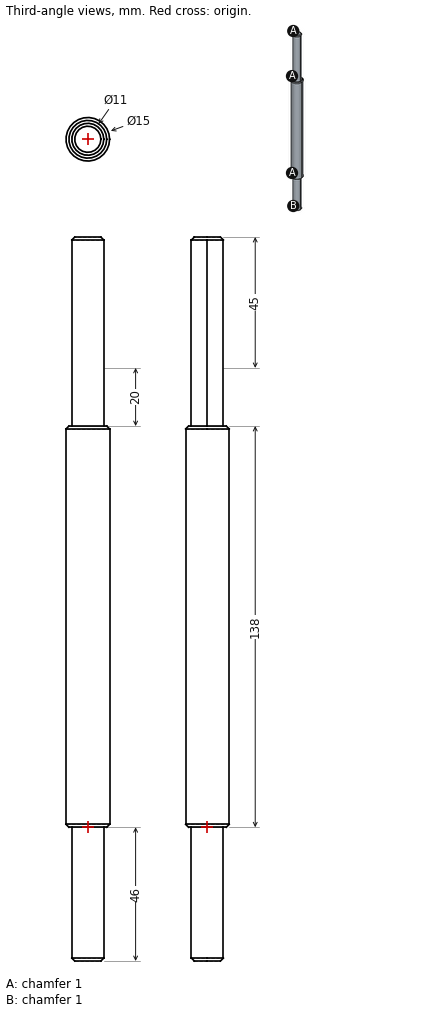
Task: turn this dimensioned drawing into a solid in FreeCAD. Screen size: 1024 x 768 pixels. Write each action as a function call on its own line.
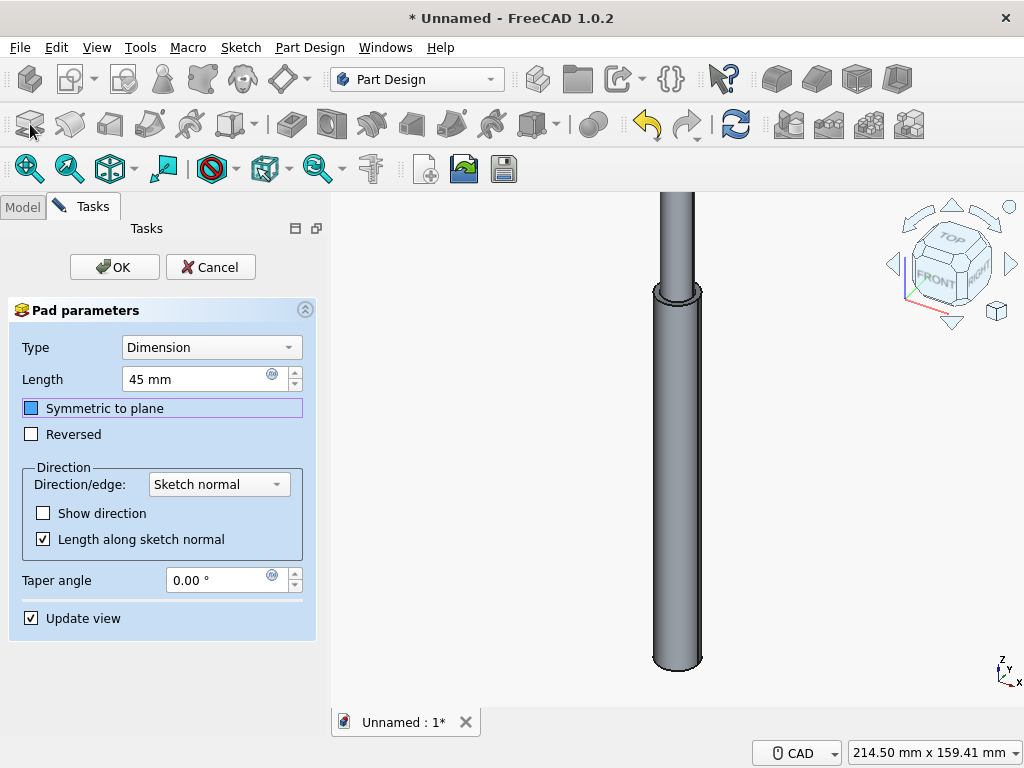
click(115, 267)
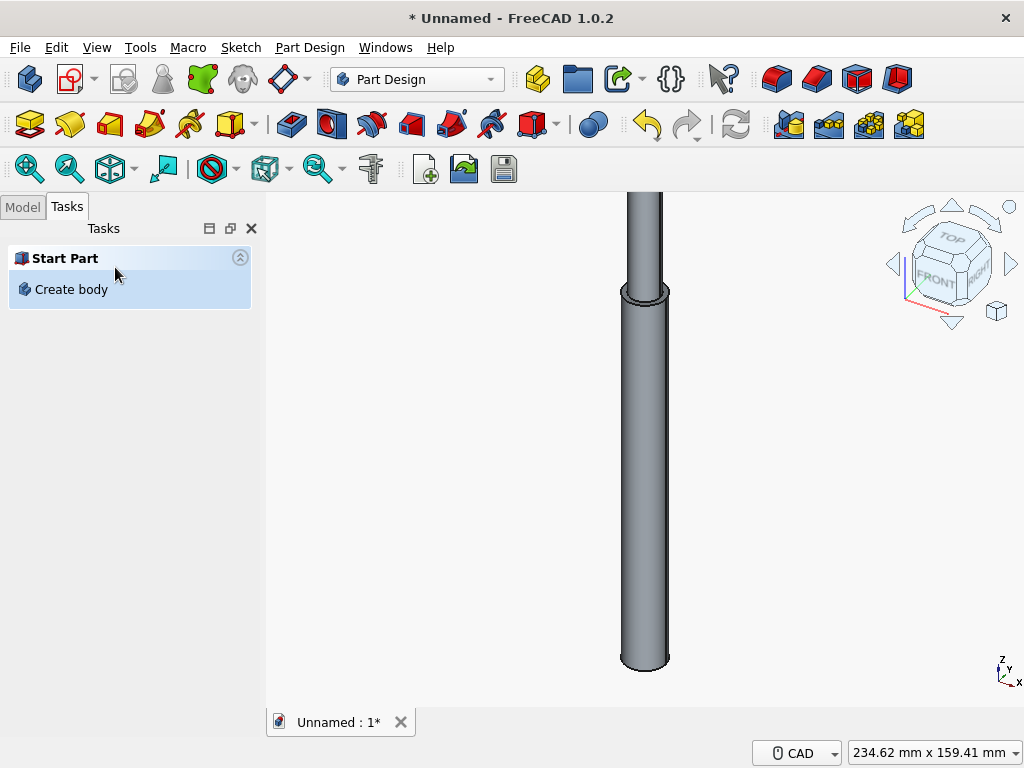
click(30, 170)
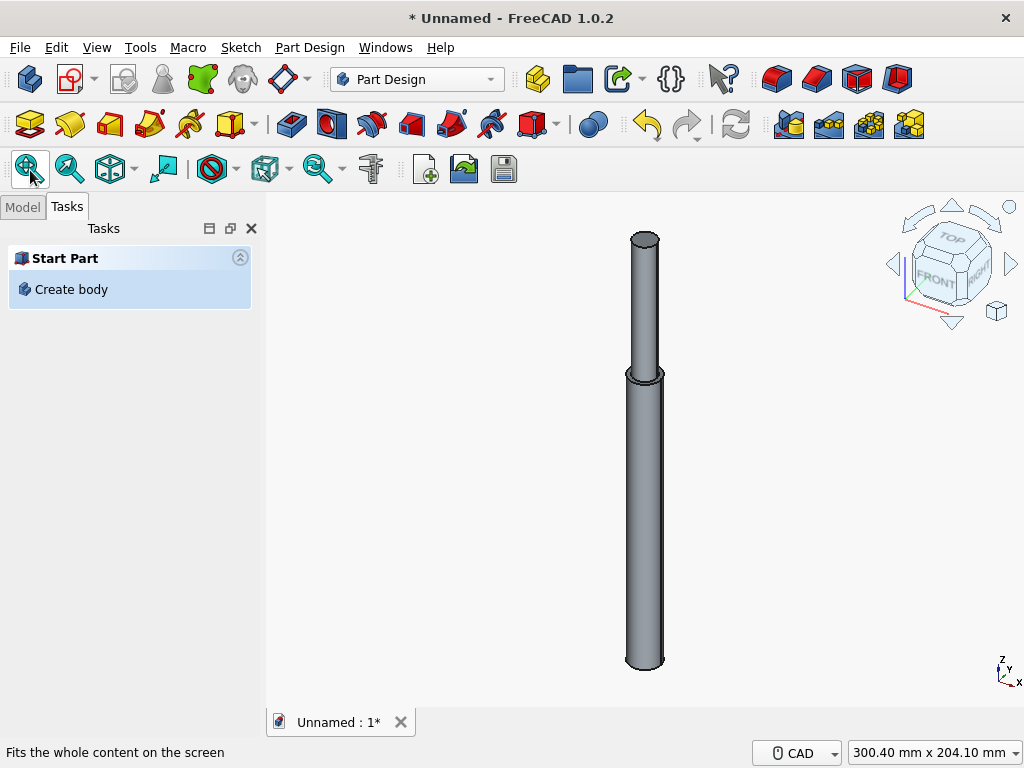
click(631, 666)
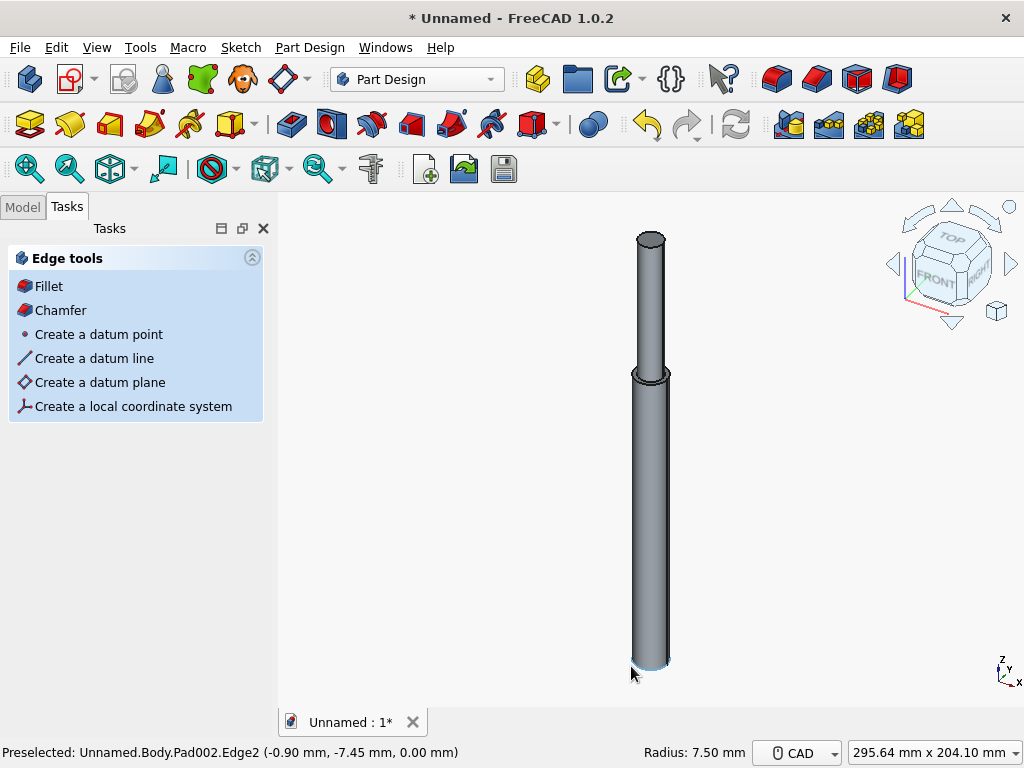
click(632, 374, ctrl)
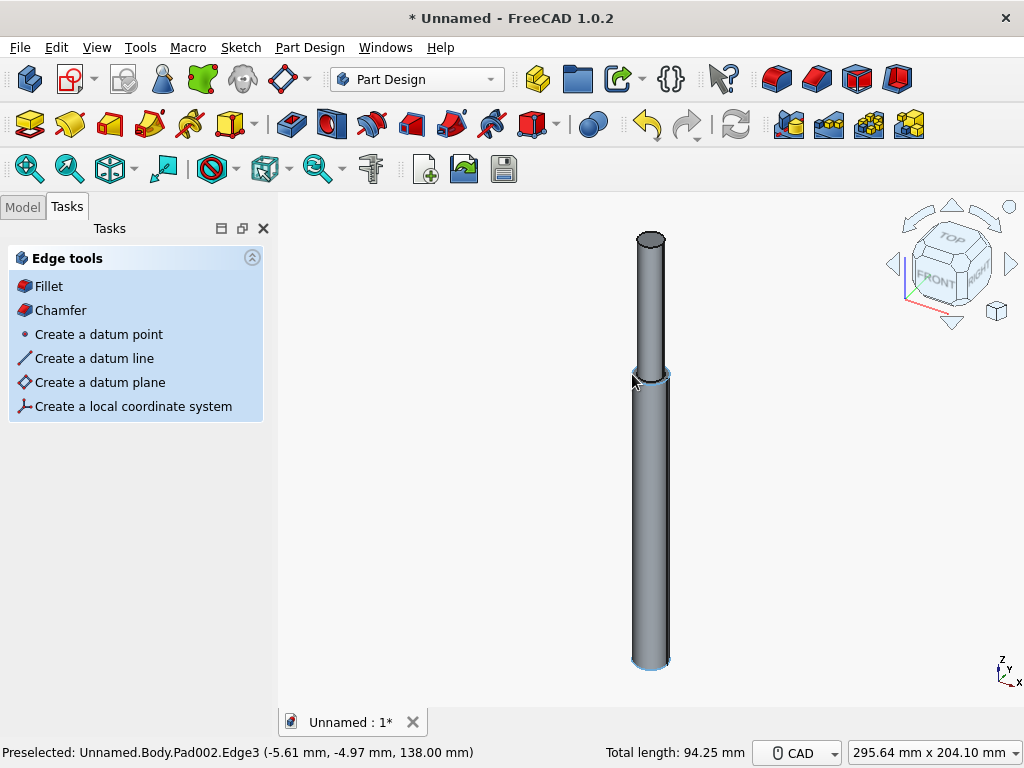
click(639, 235, ctrl)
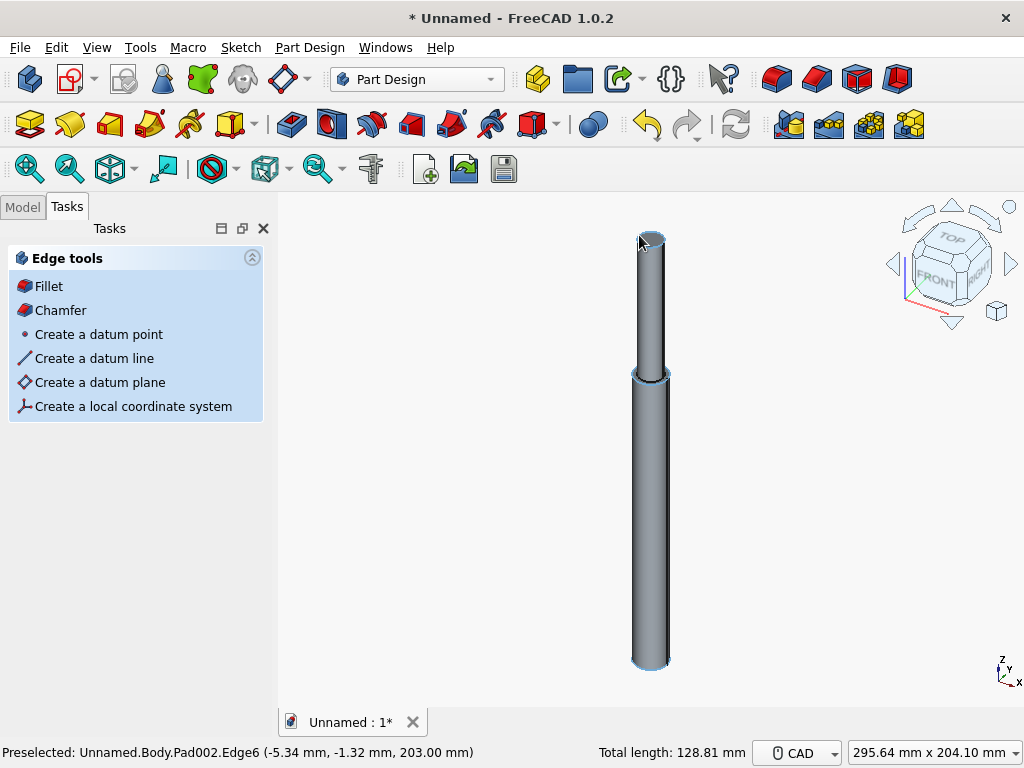
click(818, 80)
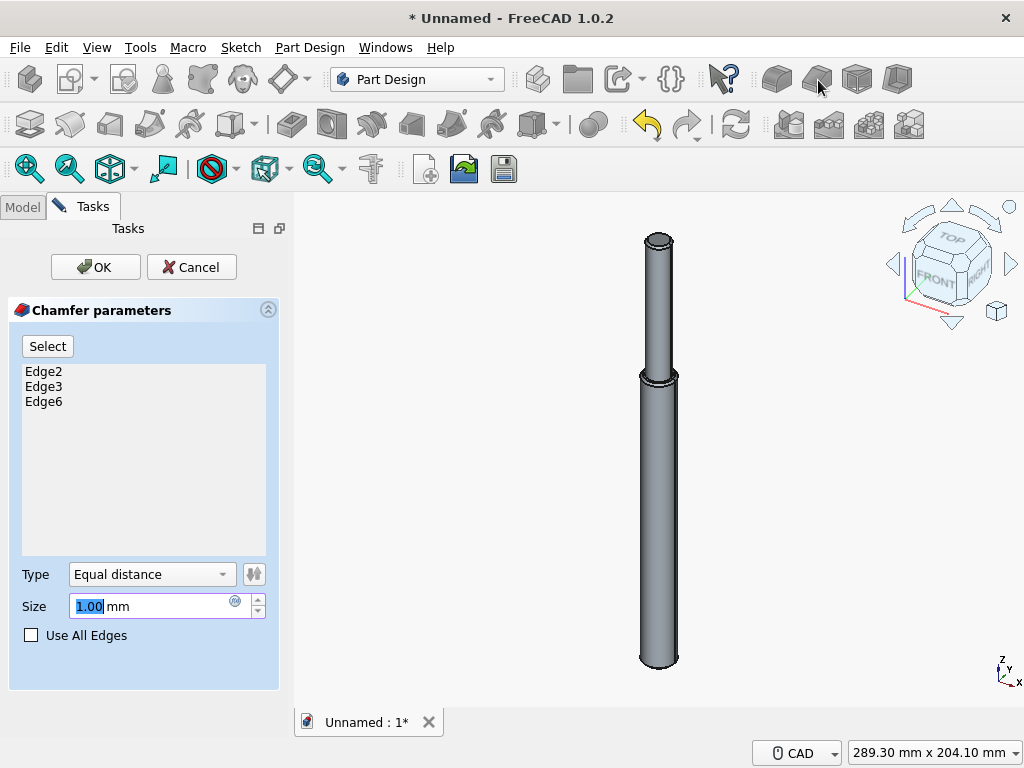
text(1)
key(Tab)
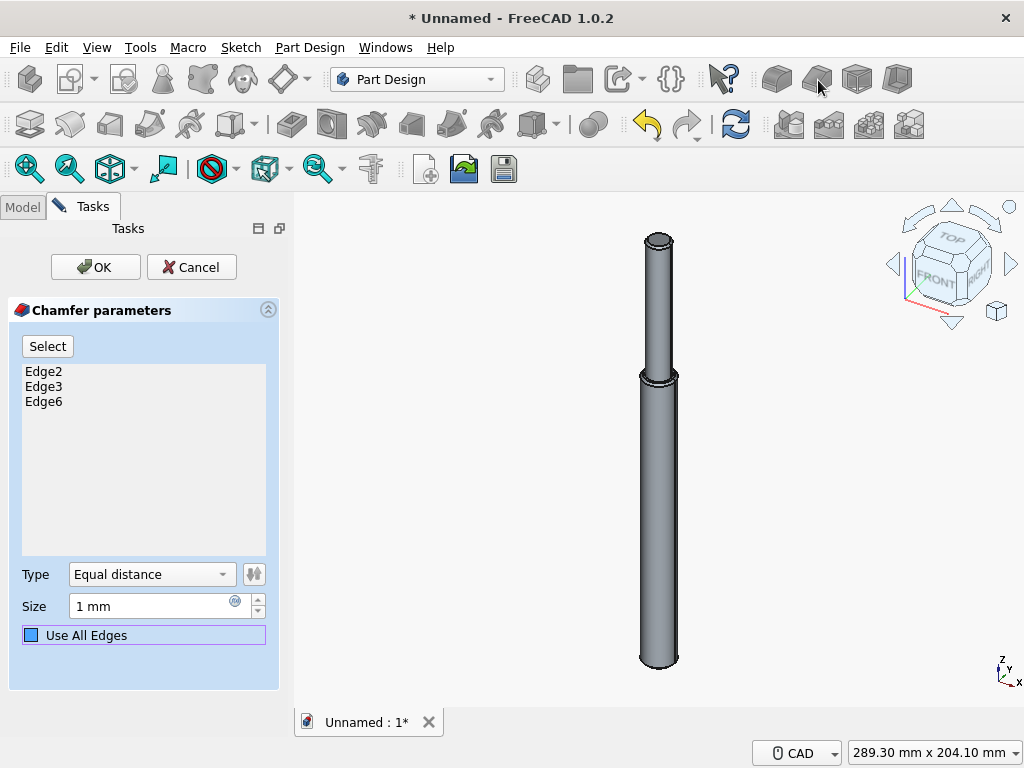
click(96, 267)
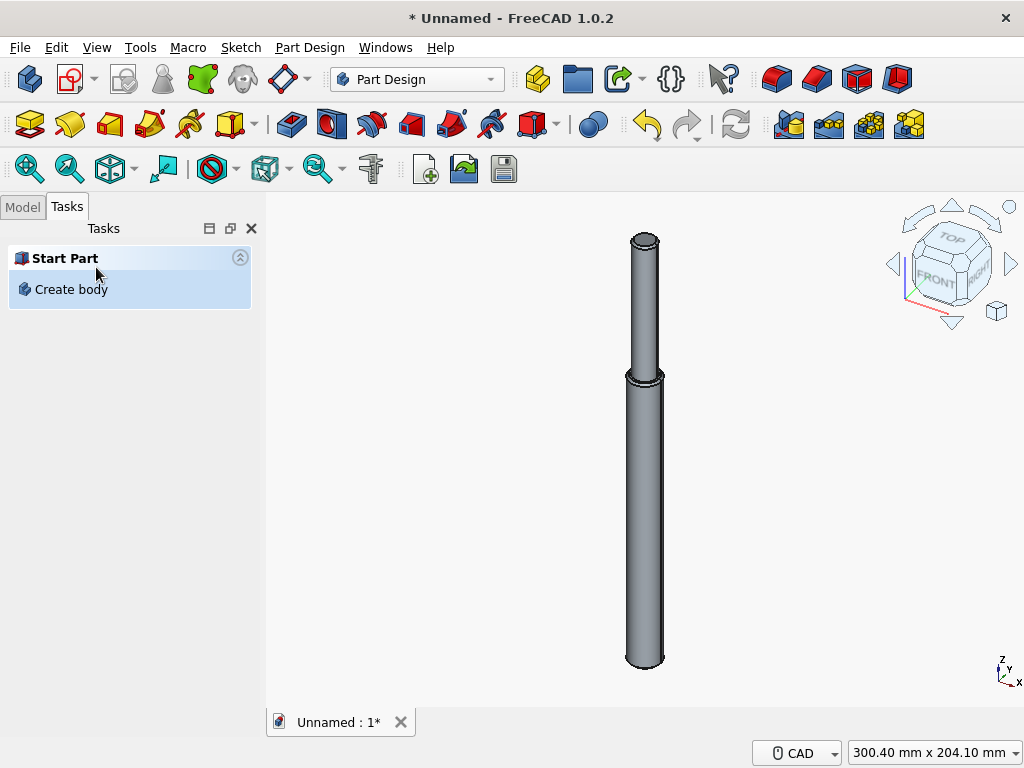
click(23, 206)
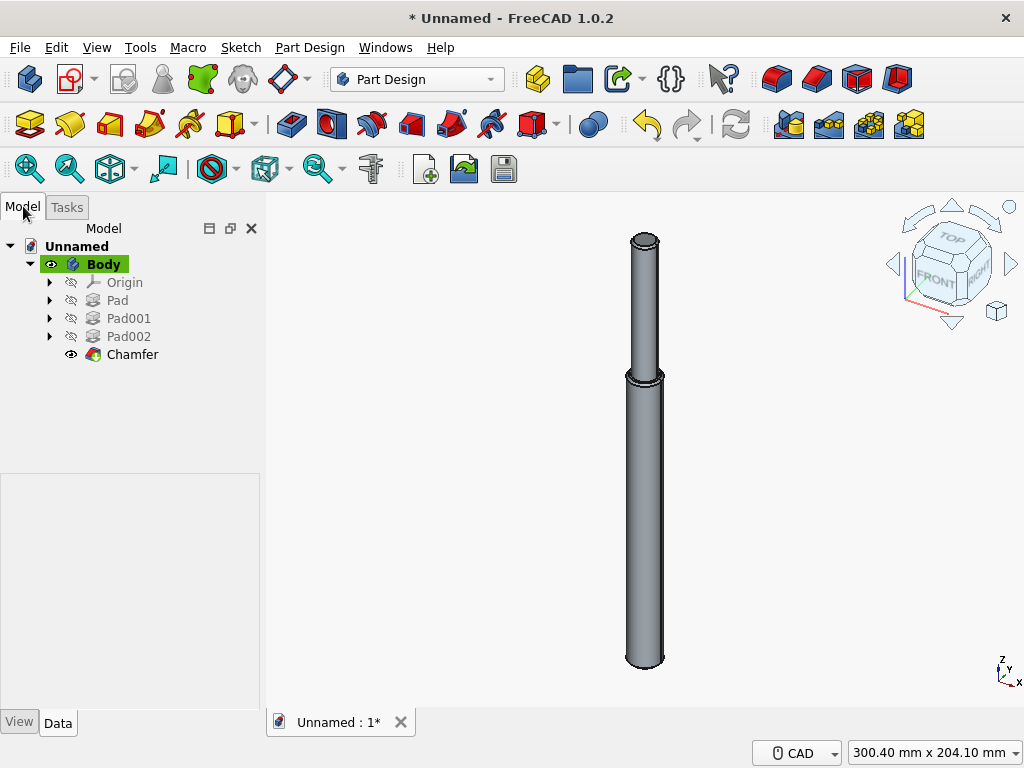
click(50, 282)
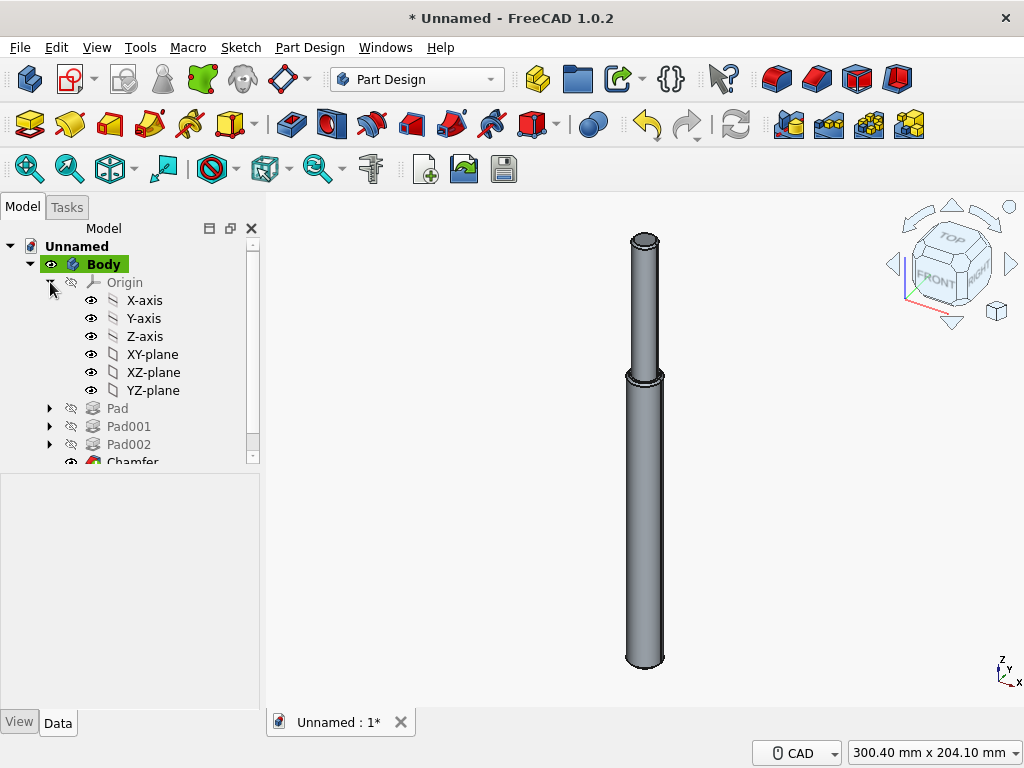
click(136, 354)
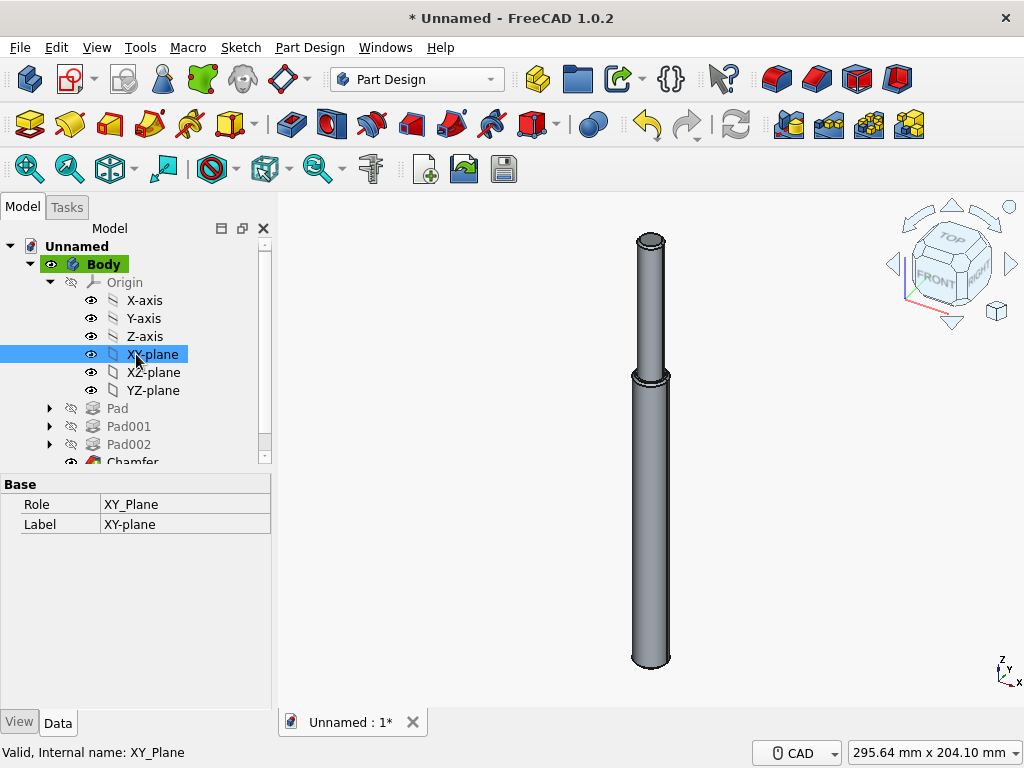
click(284, 80)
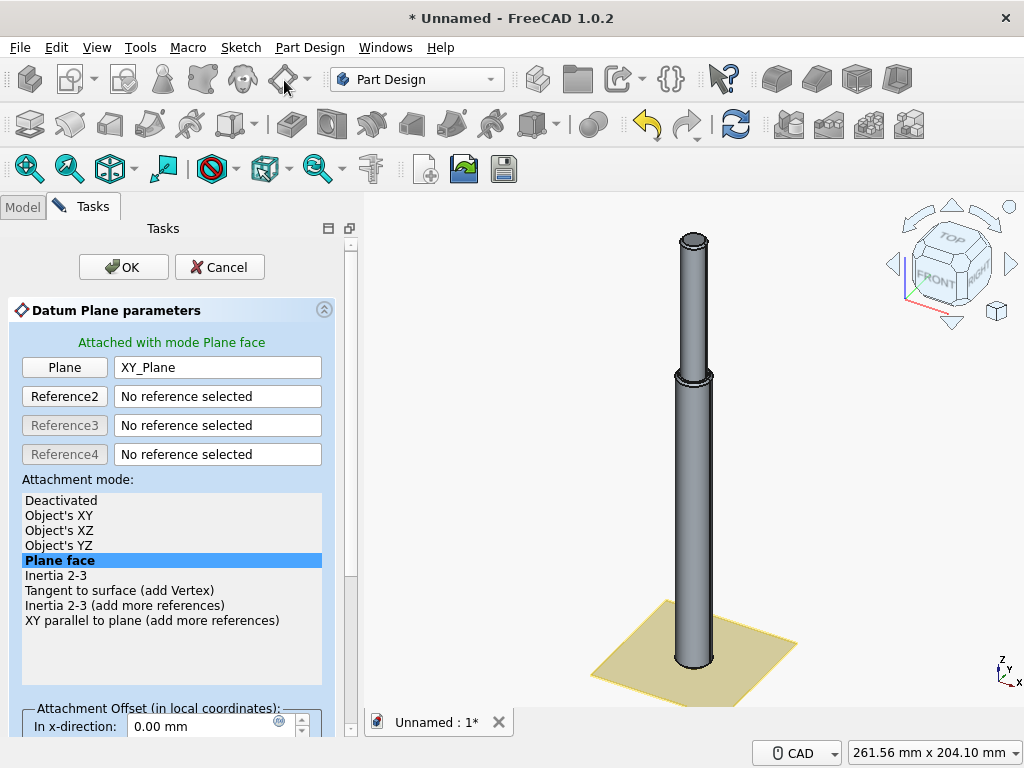
scroll(351, 487, down, 3)